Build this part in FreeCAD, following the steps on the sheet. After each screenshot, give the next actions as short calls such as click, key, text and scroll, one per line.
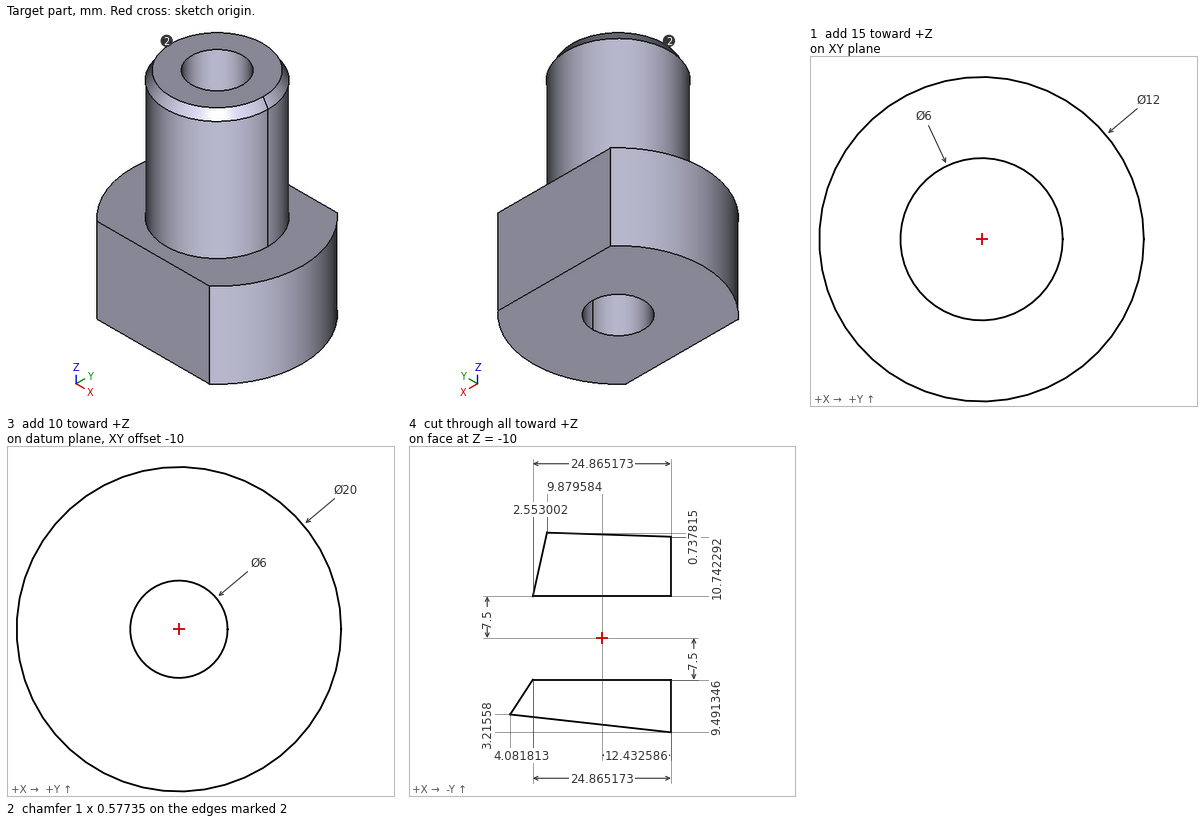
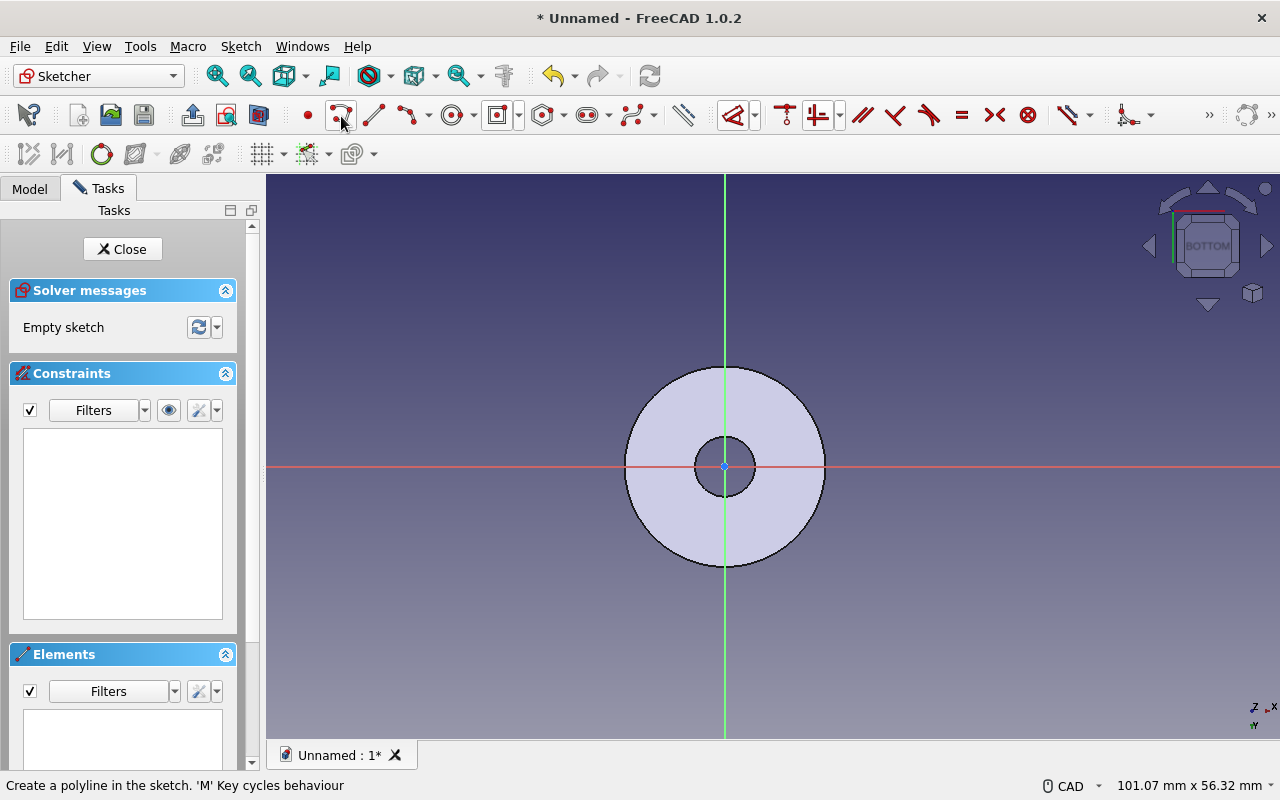
click(850, 542)
click(600, 542)
click(559, 605)
click(850, 637)
click(850, 543)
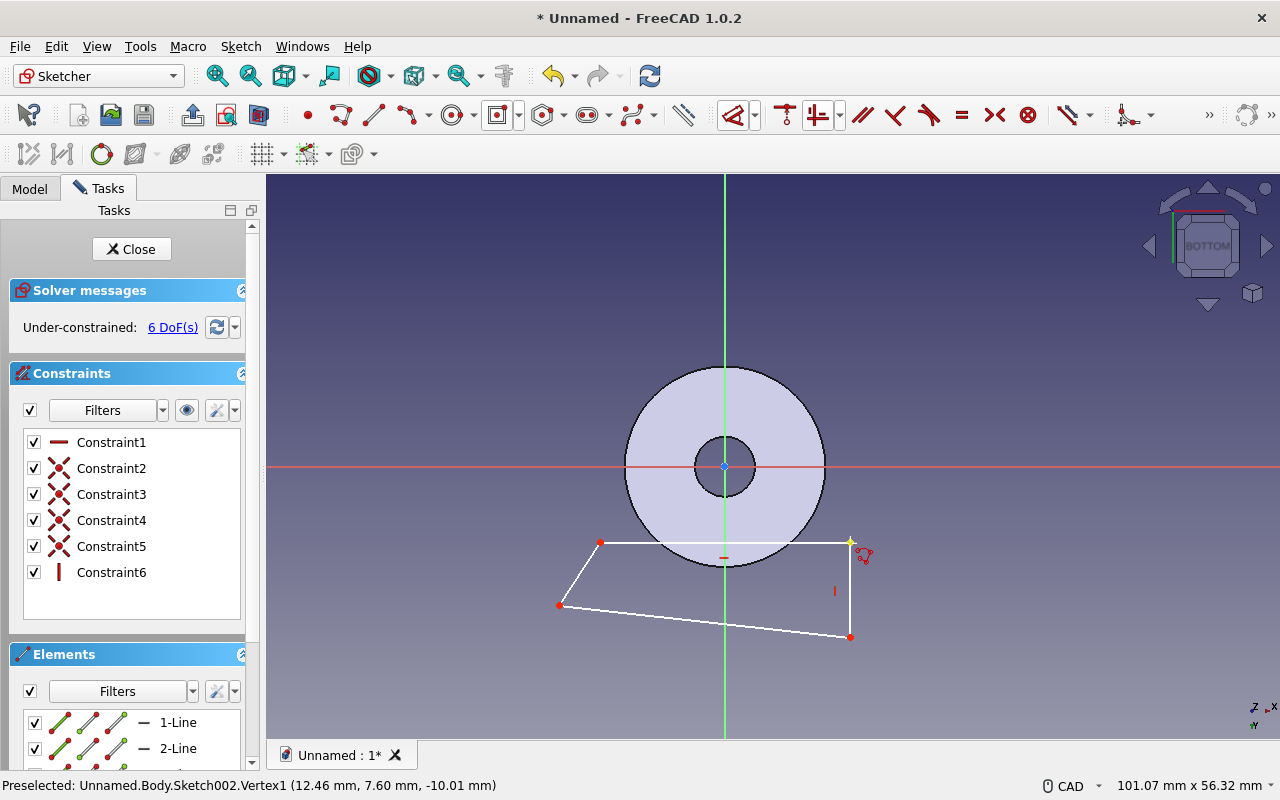
click(600, 391)
click(850, 391)
click(850, 284)
click(626, 272)
click(600, 392)
key(Escape)
key(Escape)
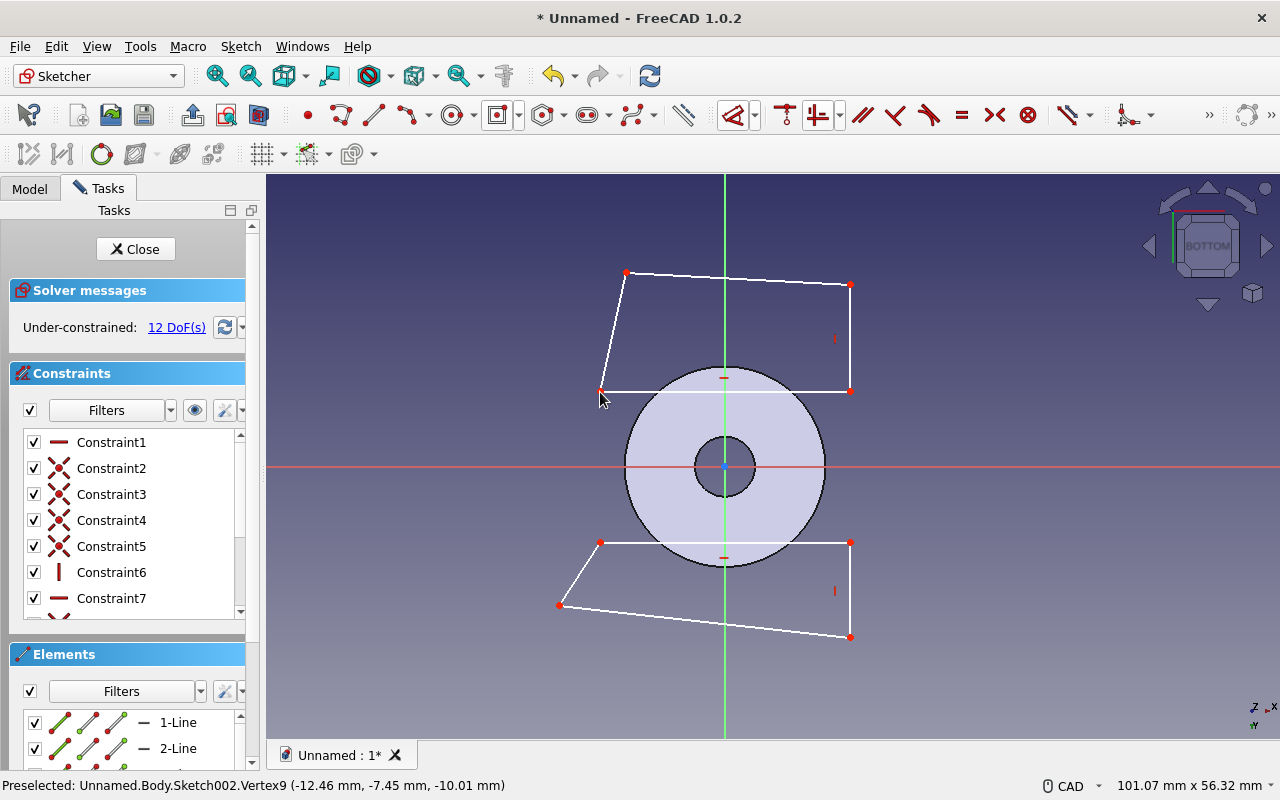
key(d)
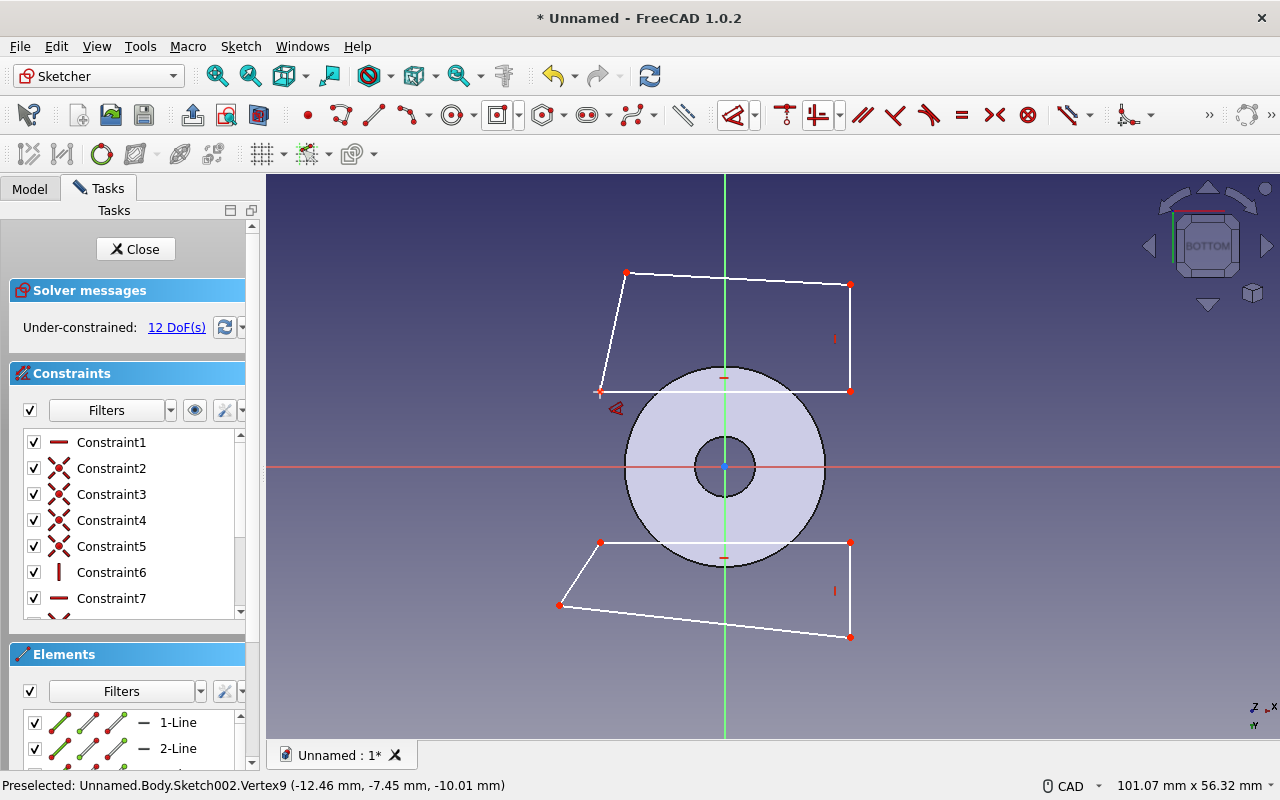
click(850, 543)
click(884, 505)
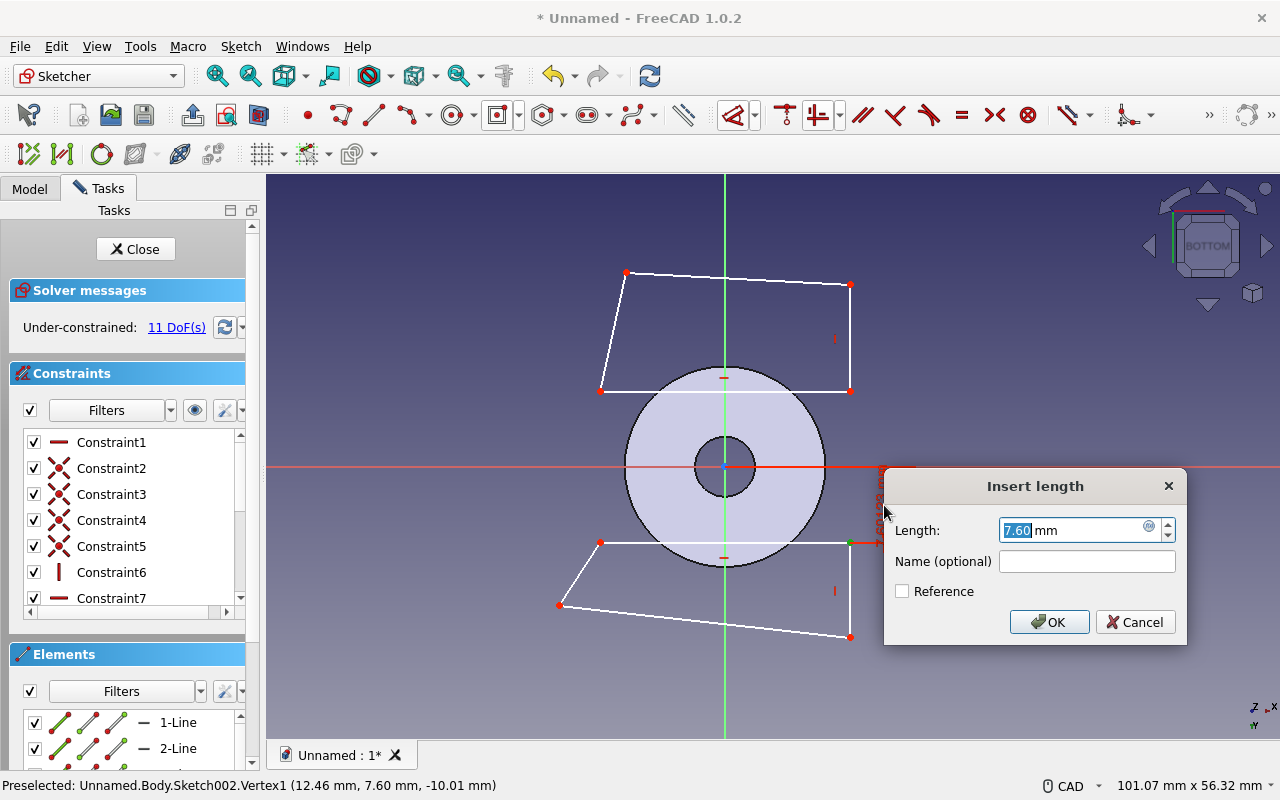
text(7.5)
key(Return)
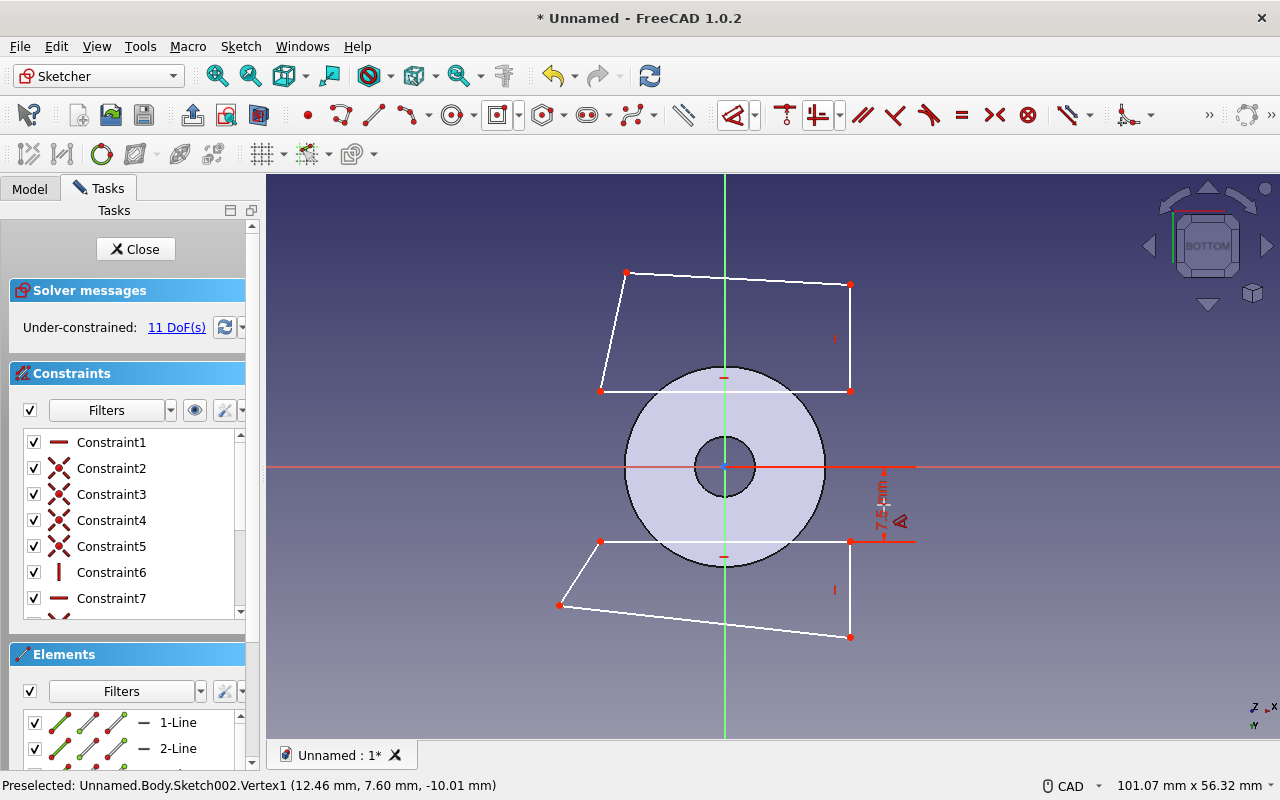
click(600, 392)
click(566, 429)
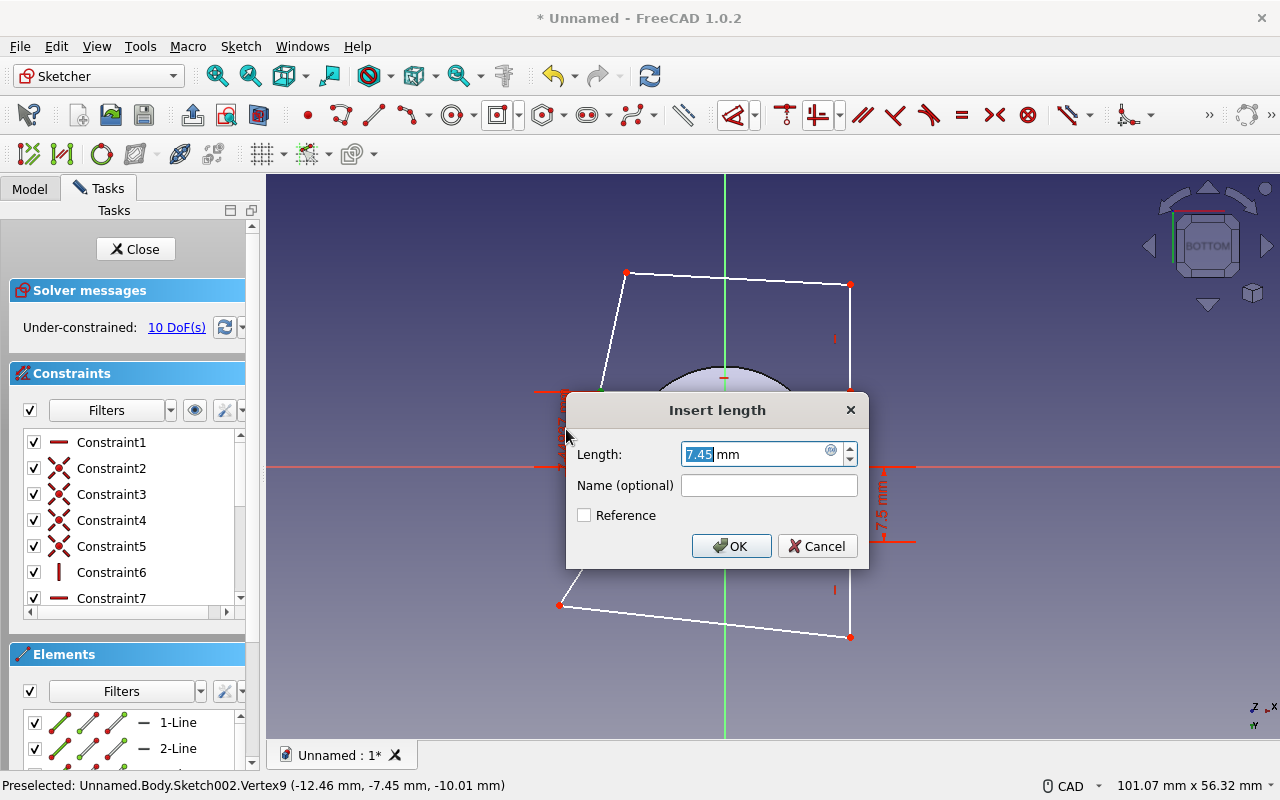
text(7.5)
key(Return)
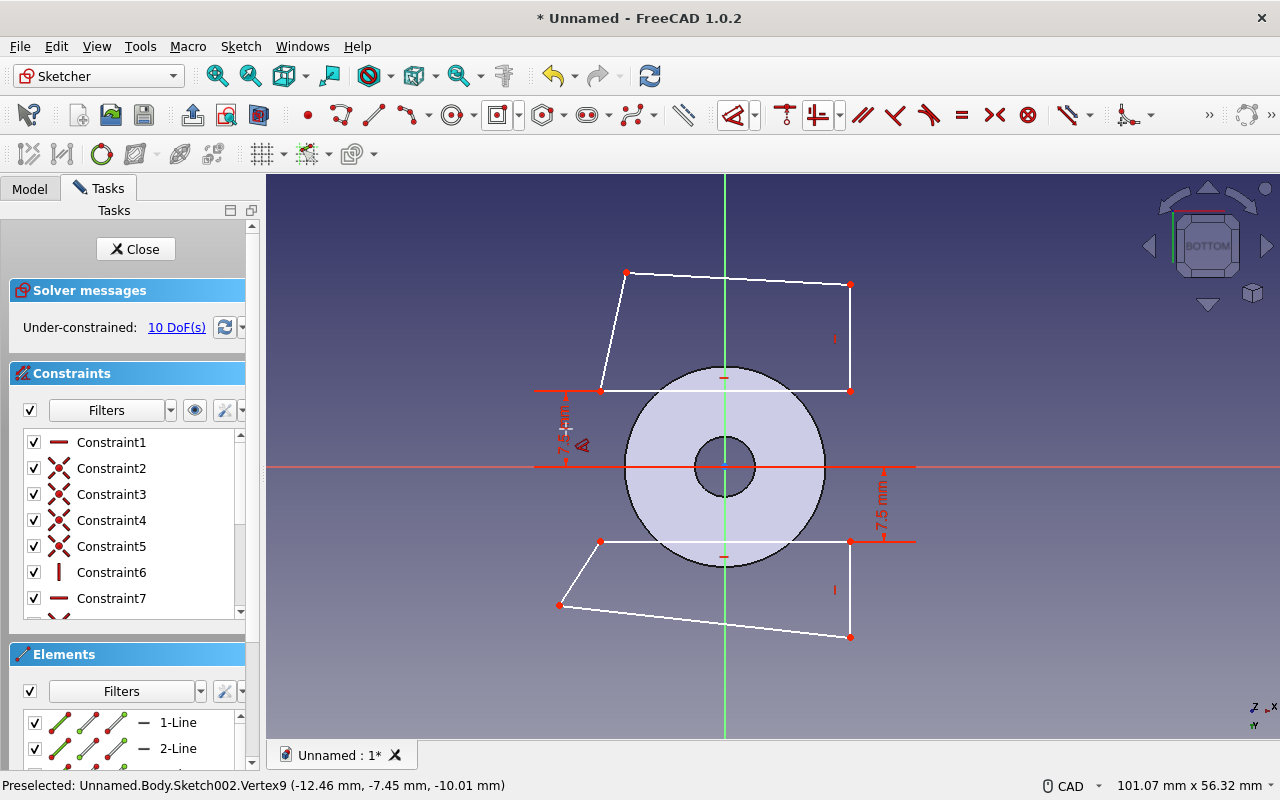
click(850, 609)
click(884, 590)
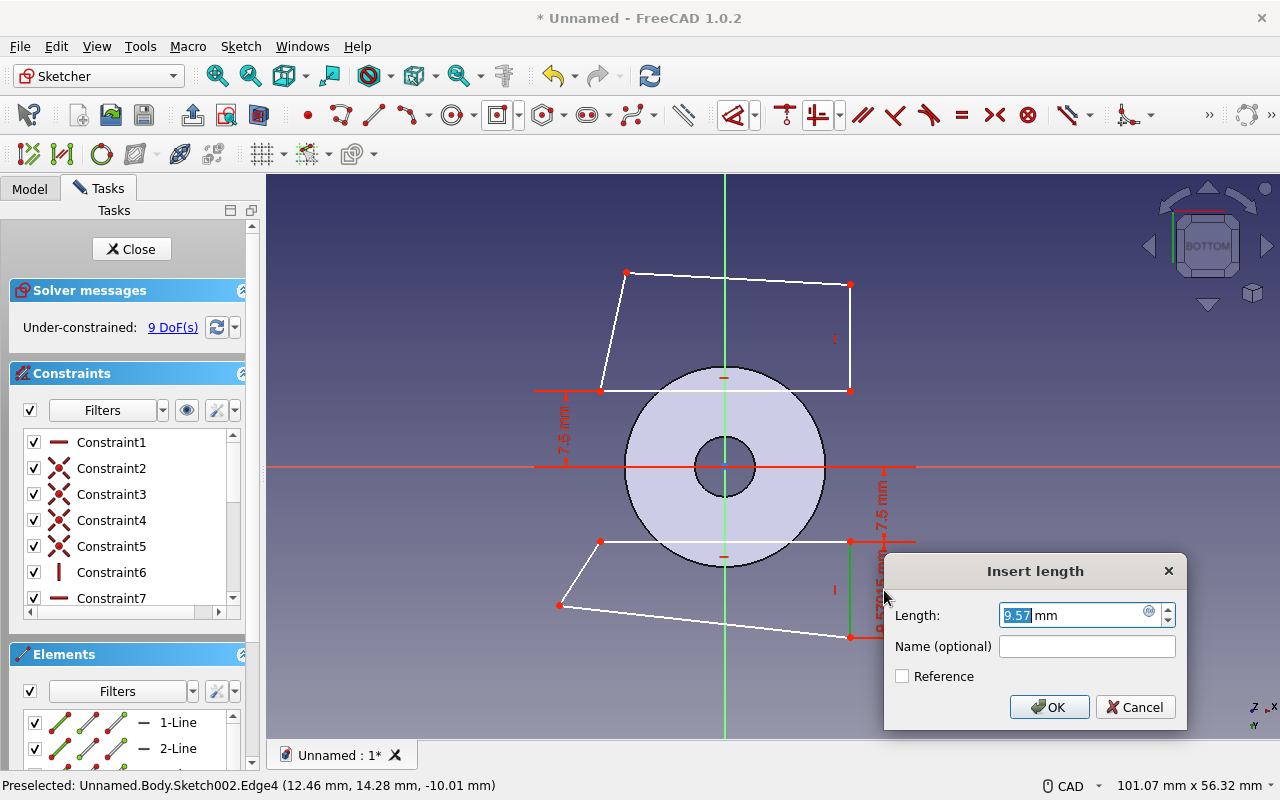
text(9.491346)
key(Return)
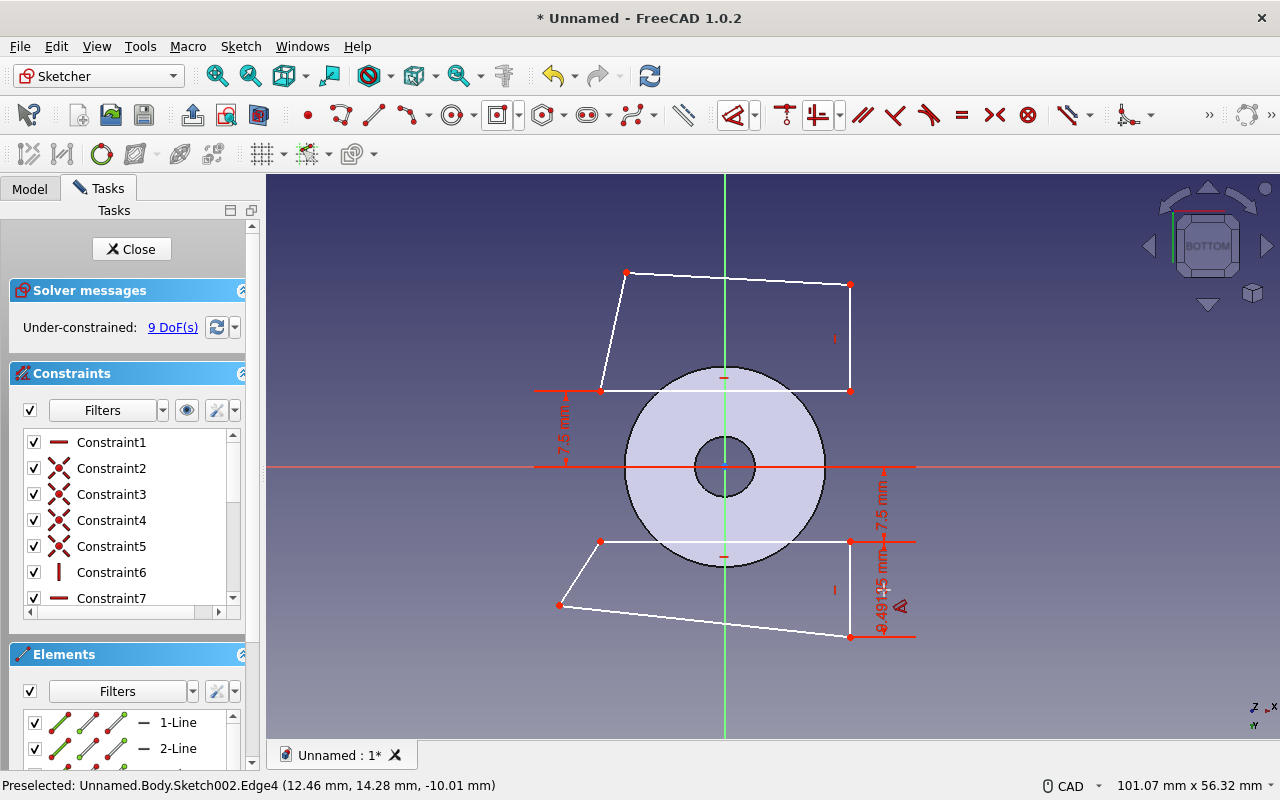
scroll(646, 615, up, 2)